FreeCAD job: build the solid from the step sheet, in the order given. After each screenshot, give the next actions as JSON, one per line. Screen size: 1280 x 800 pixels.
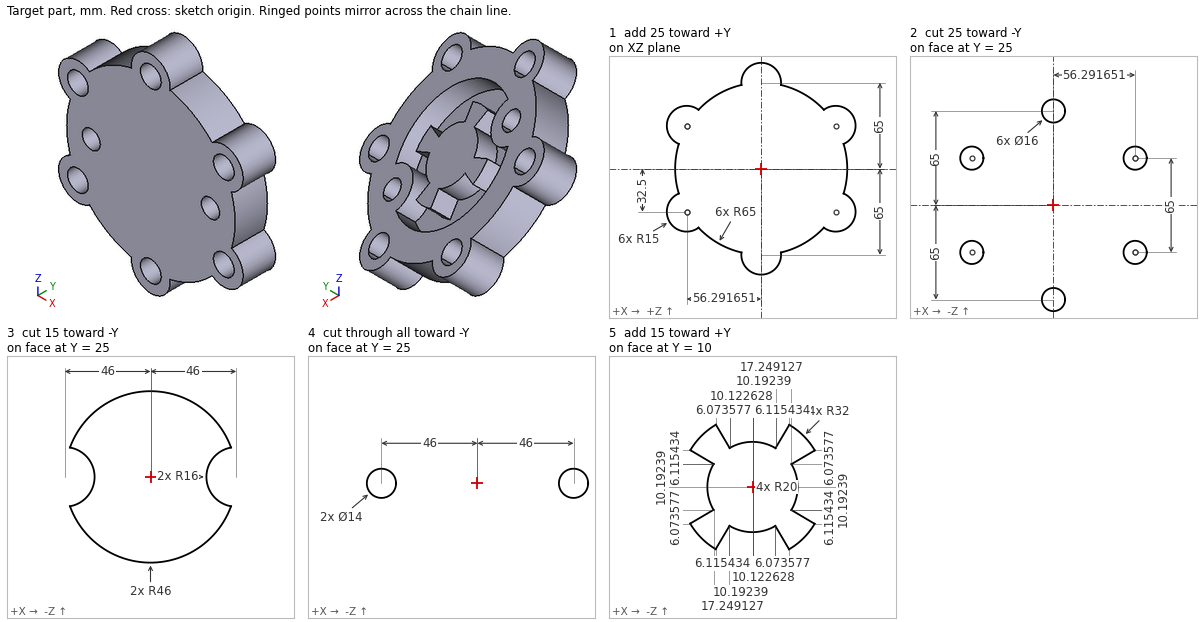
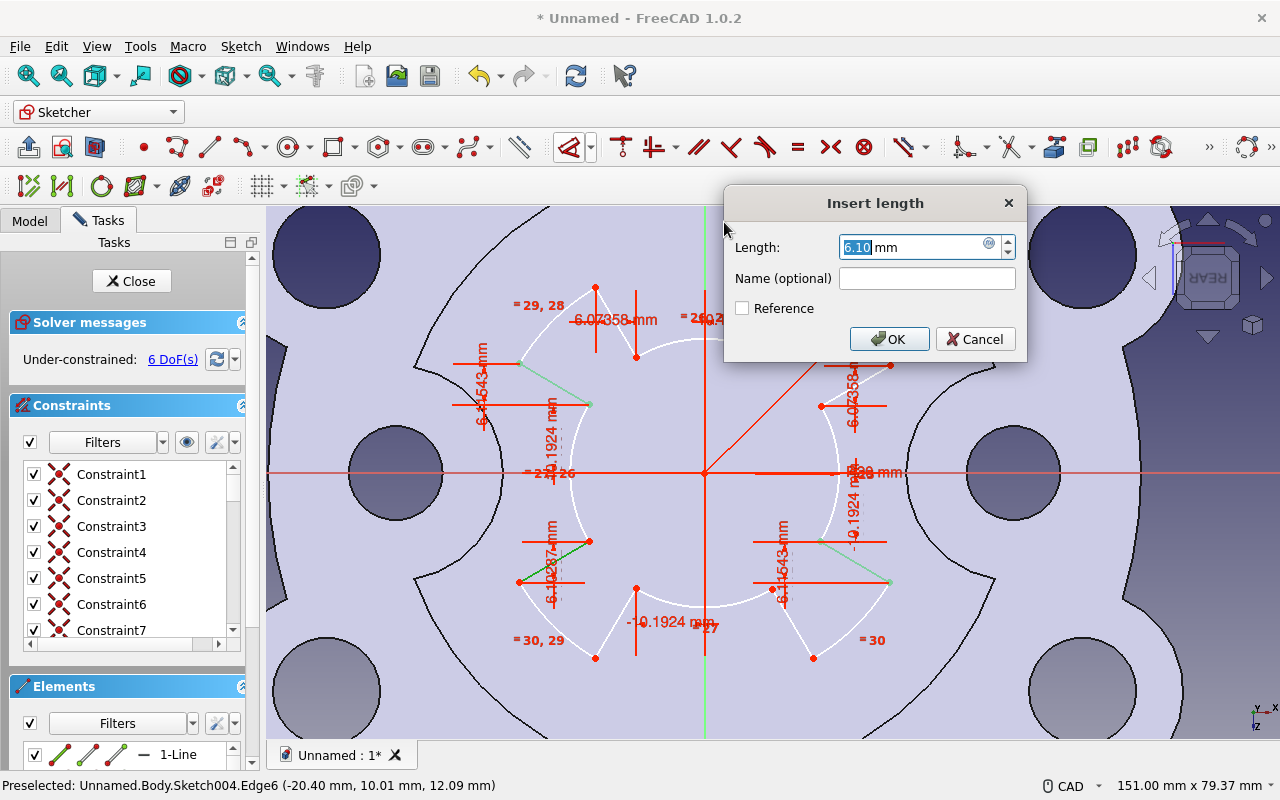
{"action": "type", "text": "6.073577"}
{"action": "key", "text": "Return"}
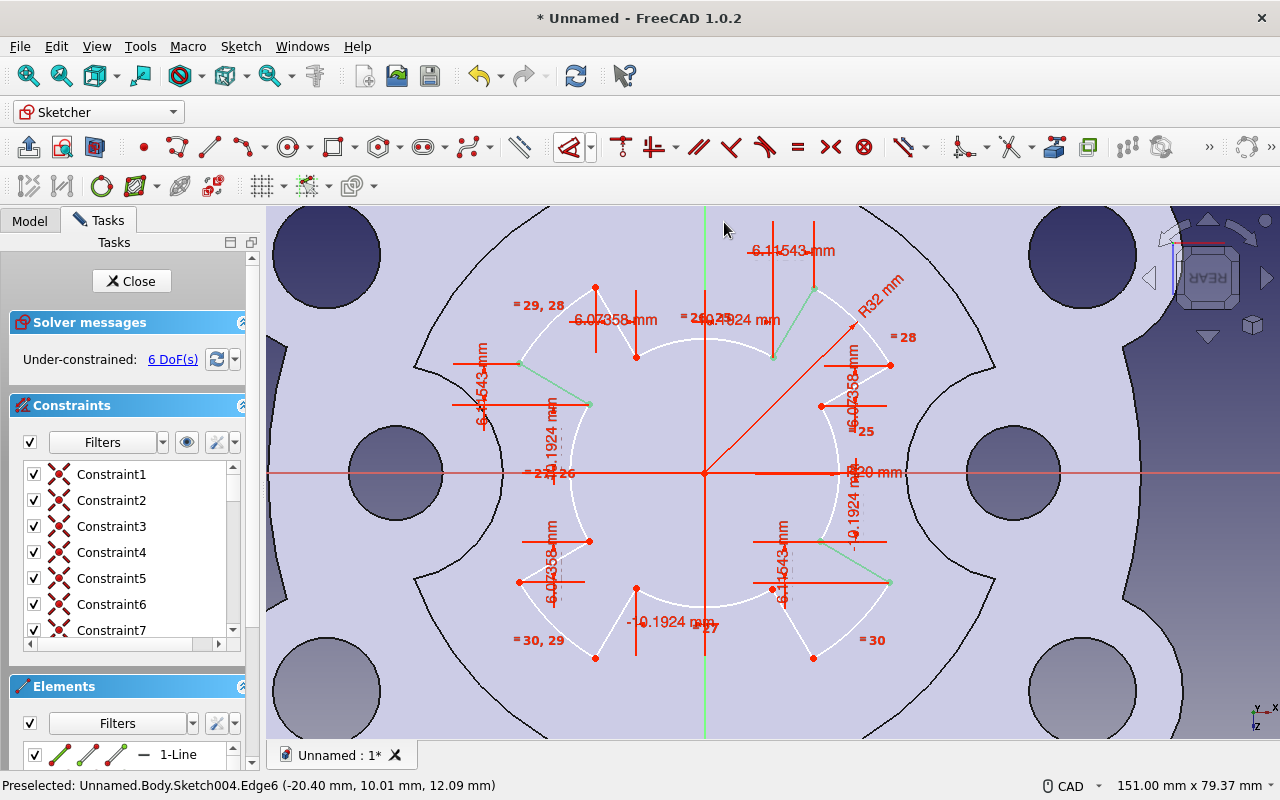
{"action": "left_click", "coordinate": [608, 637]}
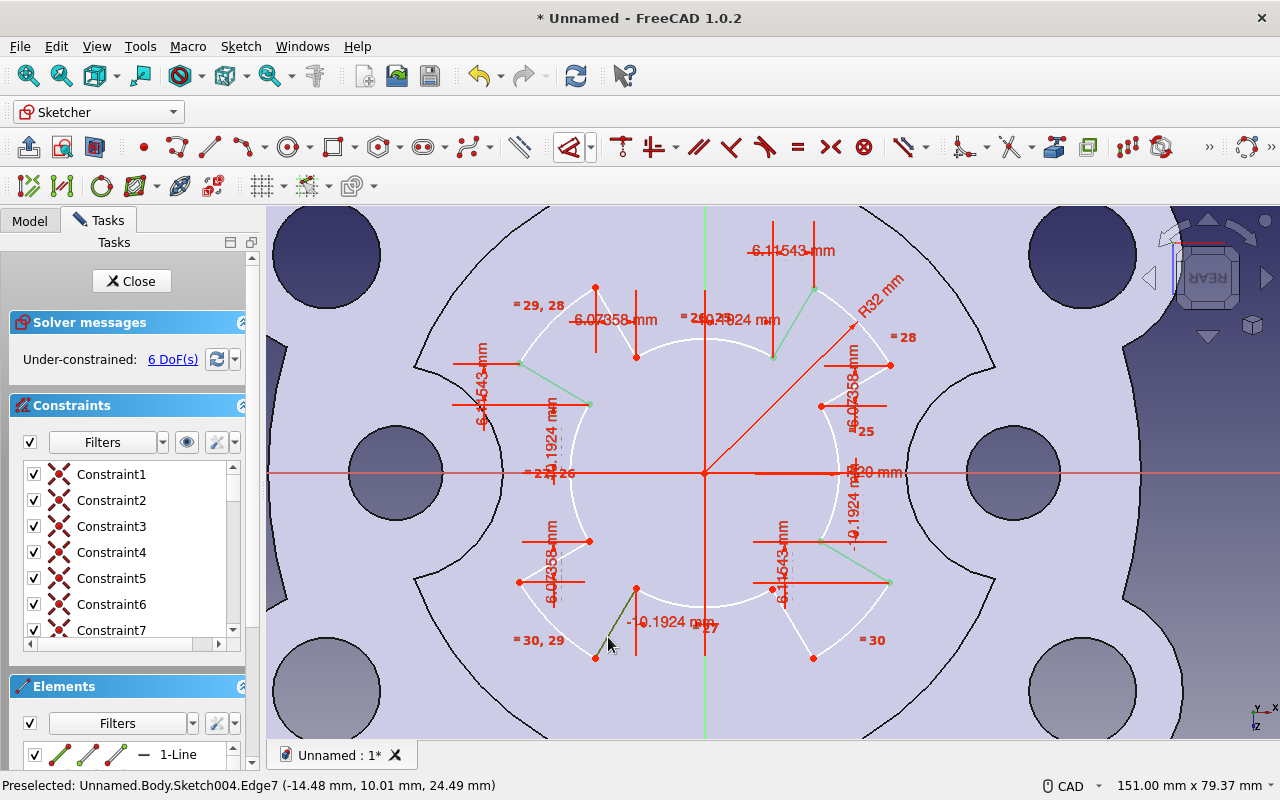
{"action": "key", "text": "l"}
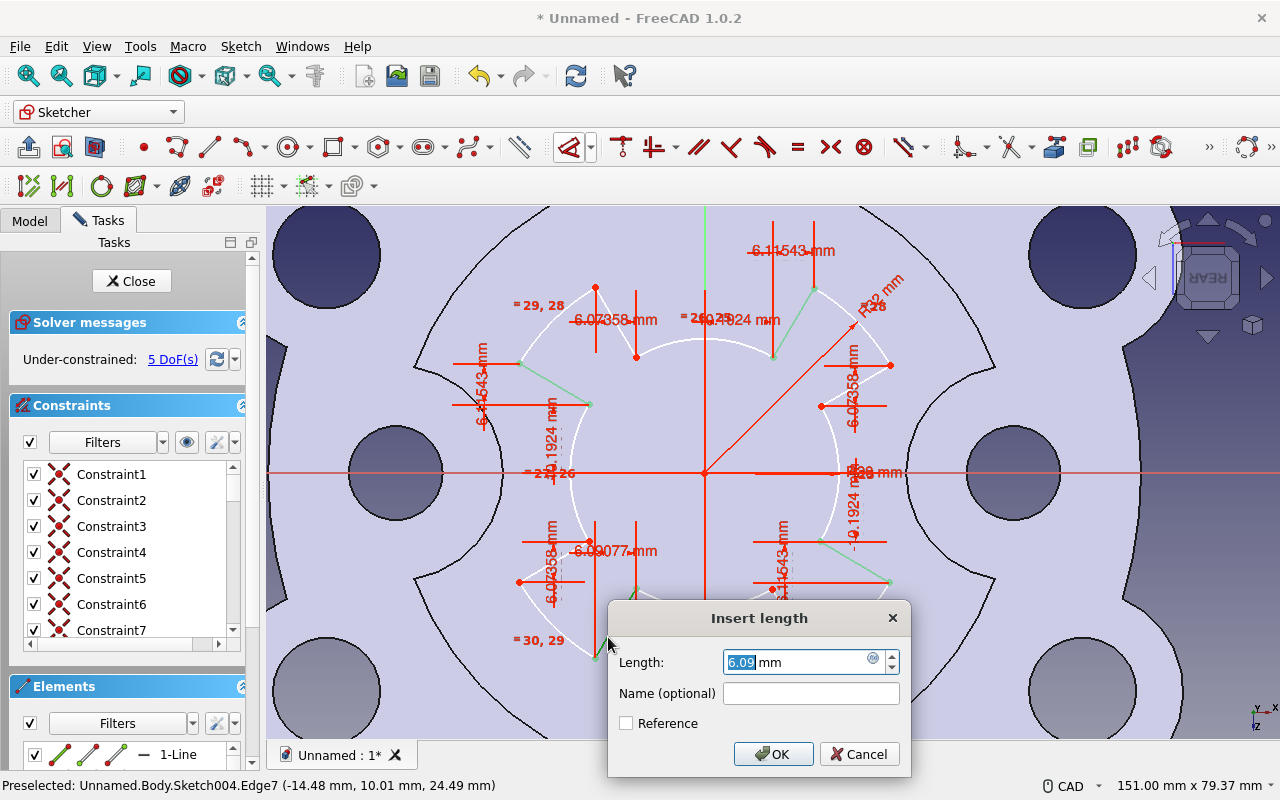
{"action": "type", "text": "6.115434"}
{"action": "key", "text": "Return"}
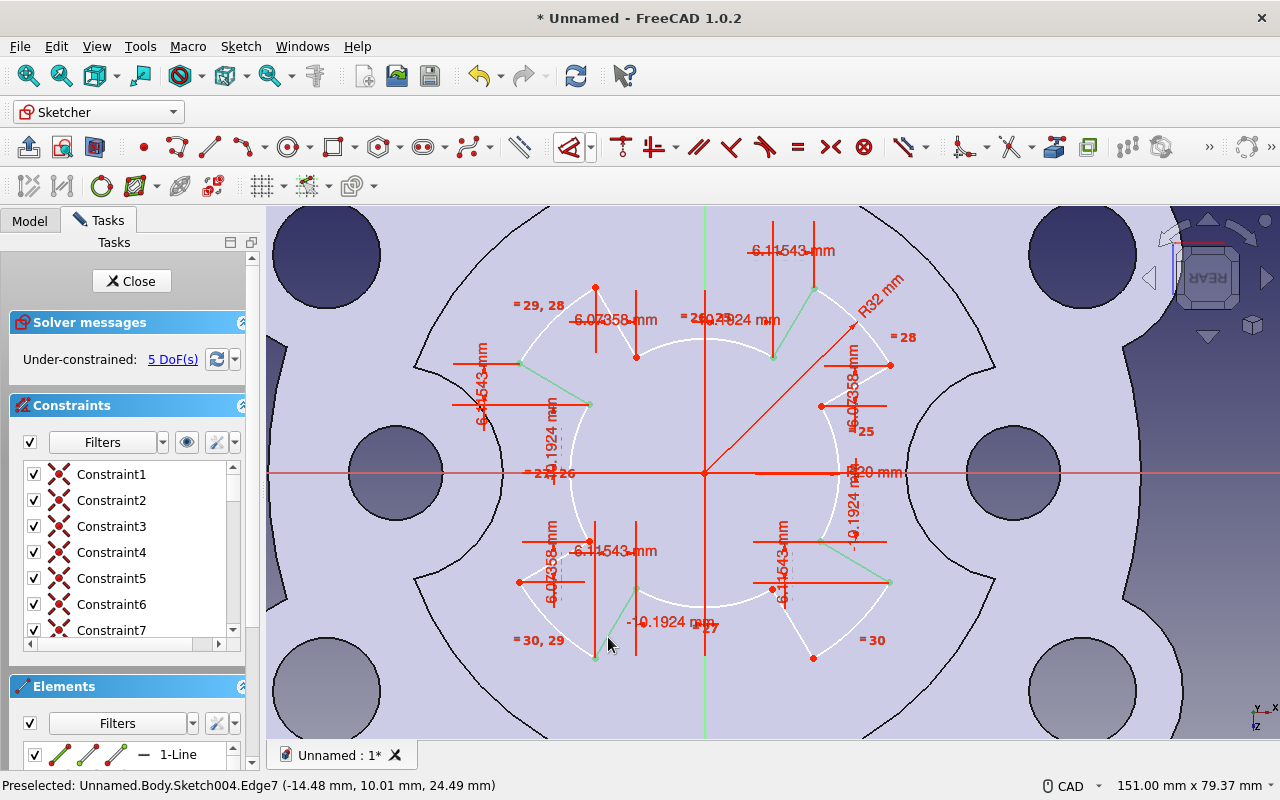
{"action": "left_click", "coordinate": [785, 610]}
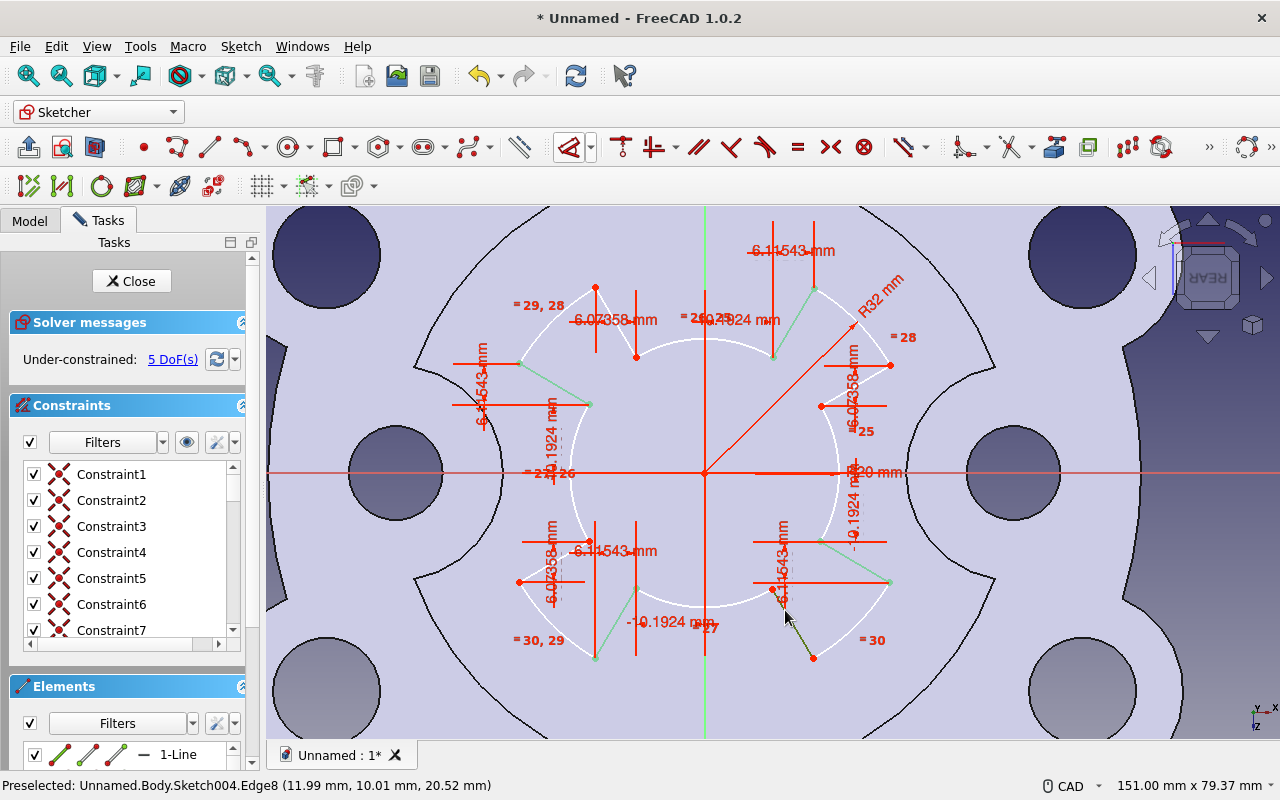
{"action": "left_click", "coordinate": [590, 148]}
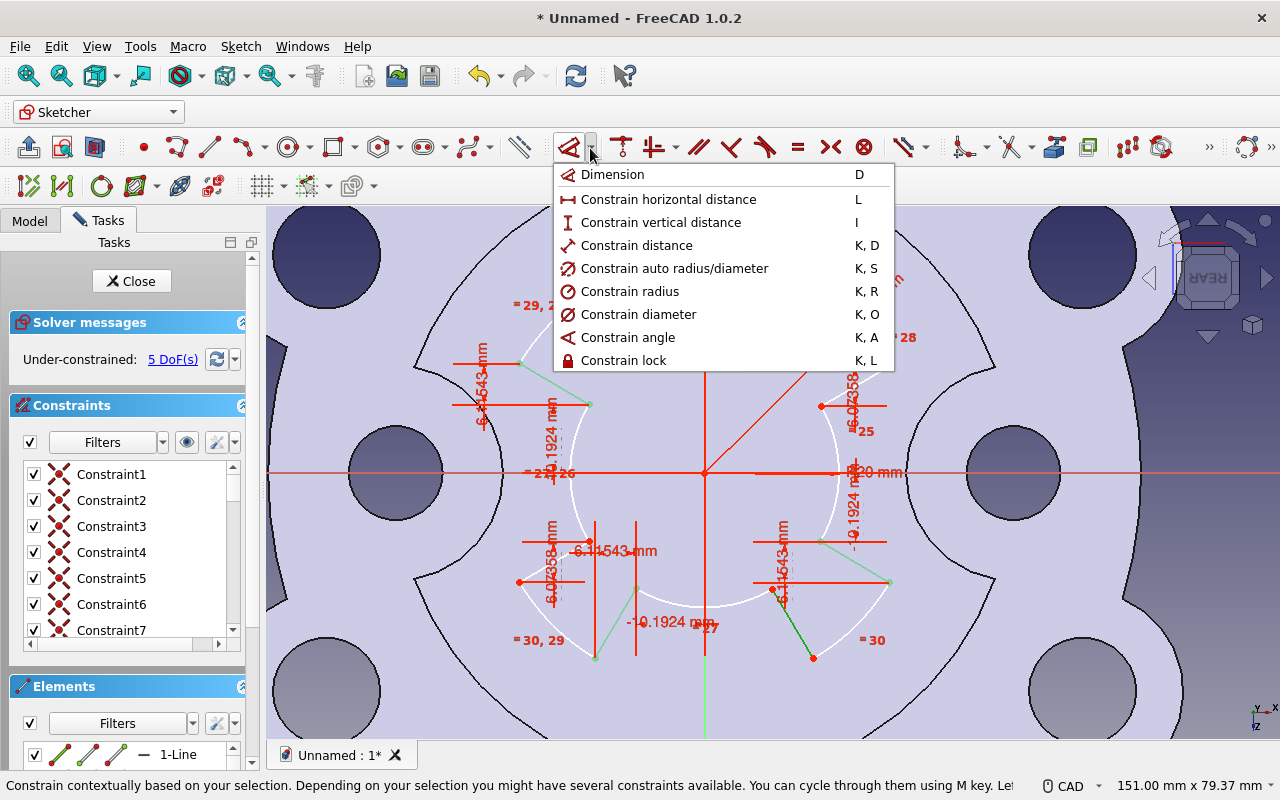
{"action": "left_click", "coordinate": [724, 200]}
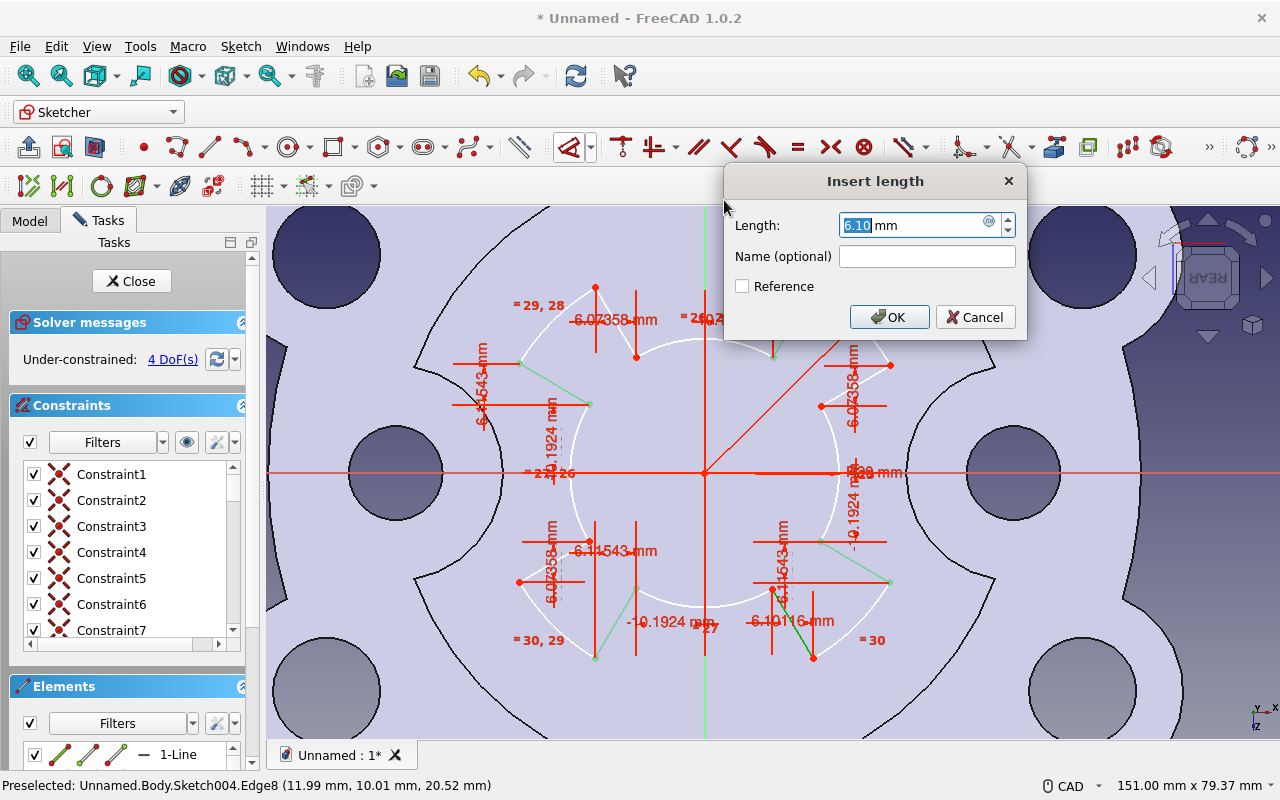
{"action": "type", "text": "6.073577"}
{"action": "key", "text": "Return"}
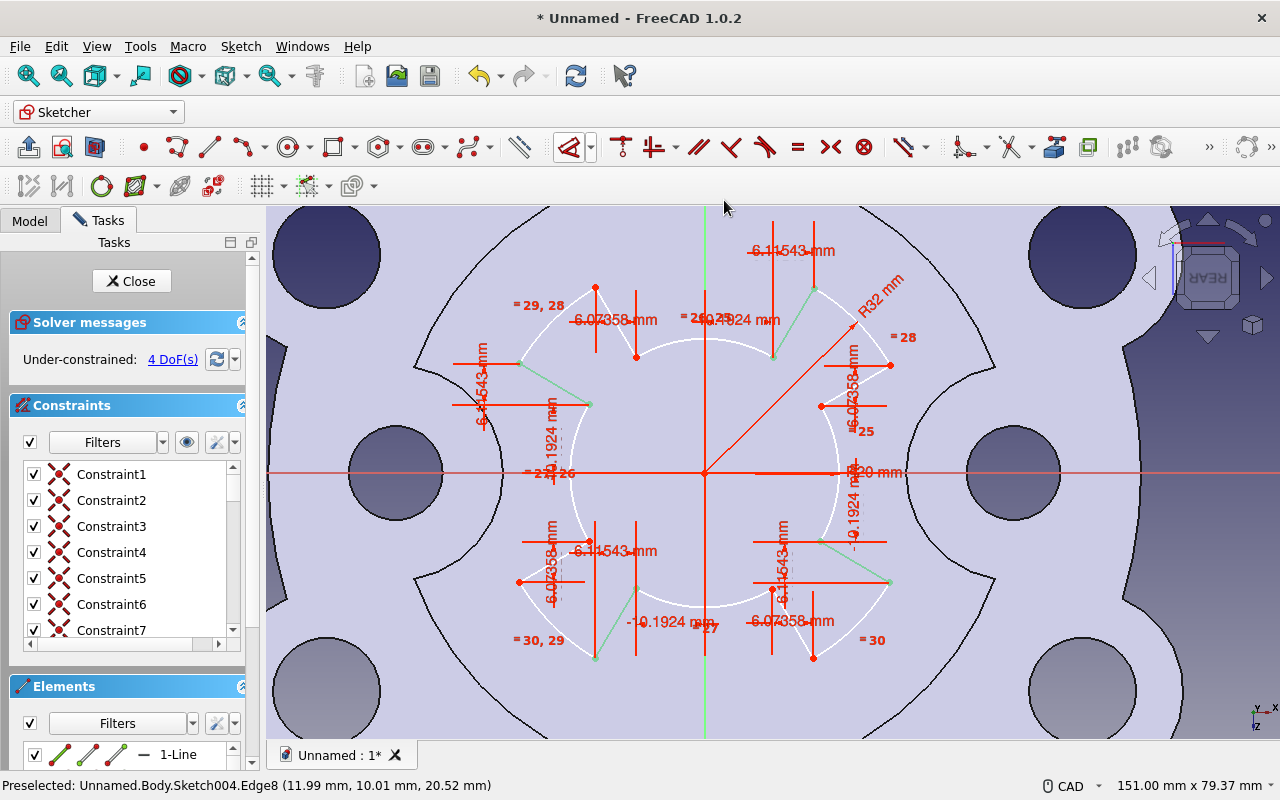
{"action": "left_click", "coordinate": [821, 406]}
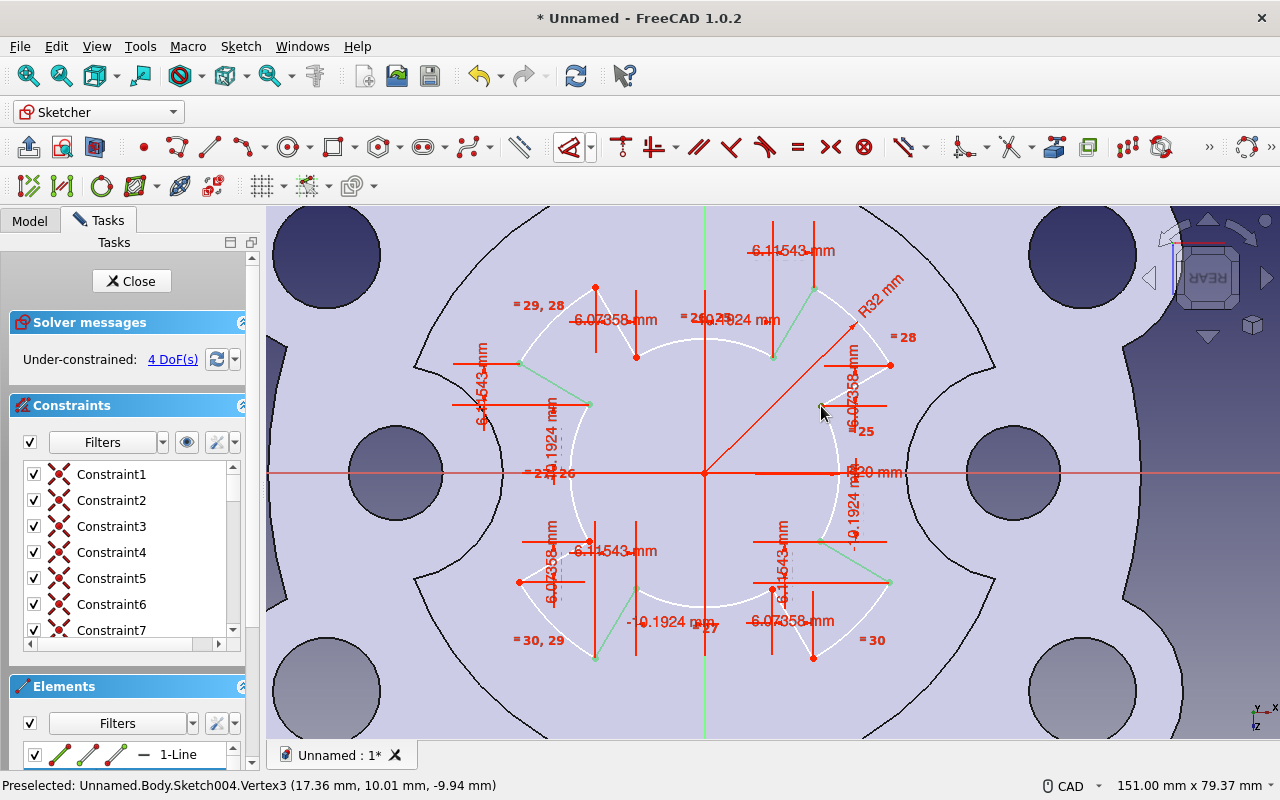
{"action": "left_click", "coordinate": [590, 148]}